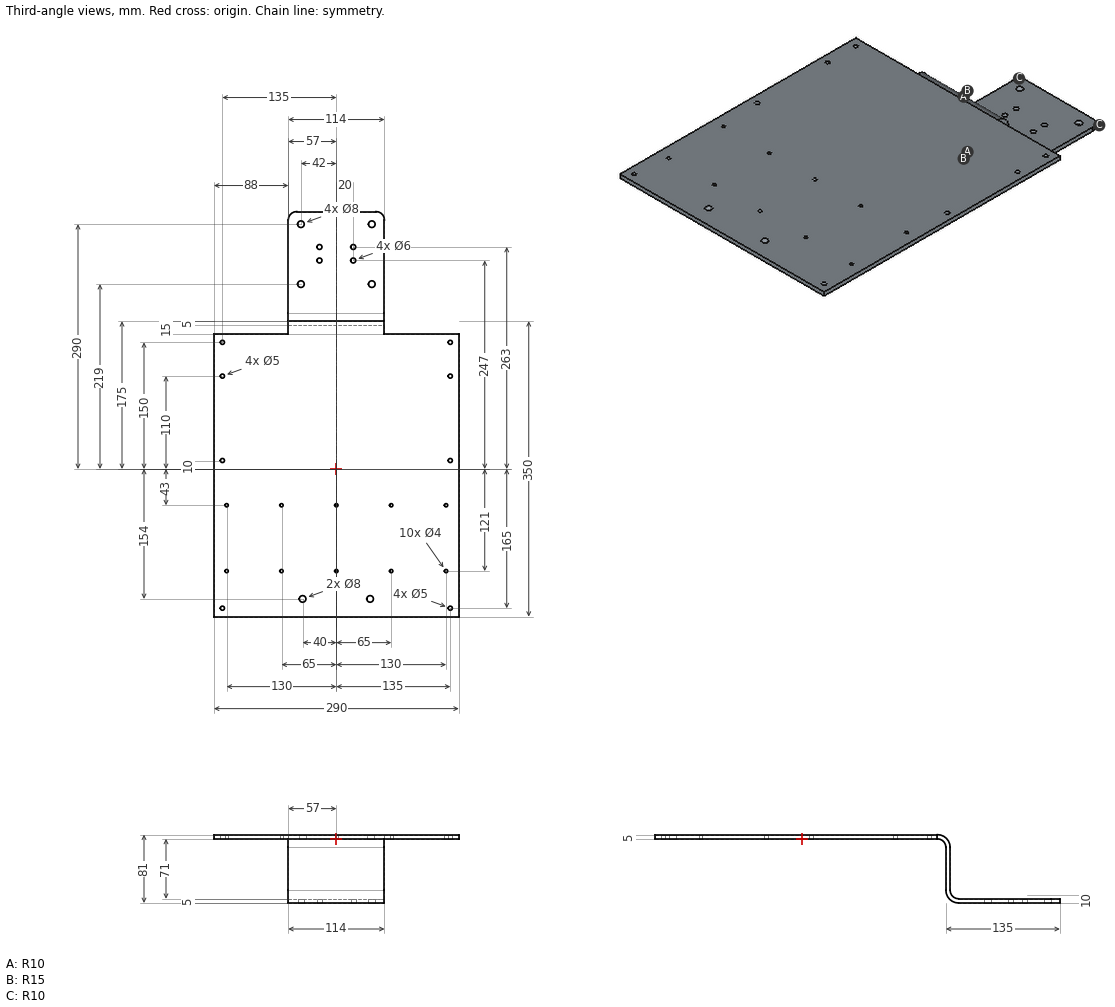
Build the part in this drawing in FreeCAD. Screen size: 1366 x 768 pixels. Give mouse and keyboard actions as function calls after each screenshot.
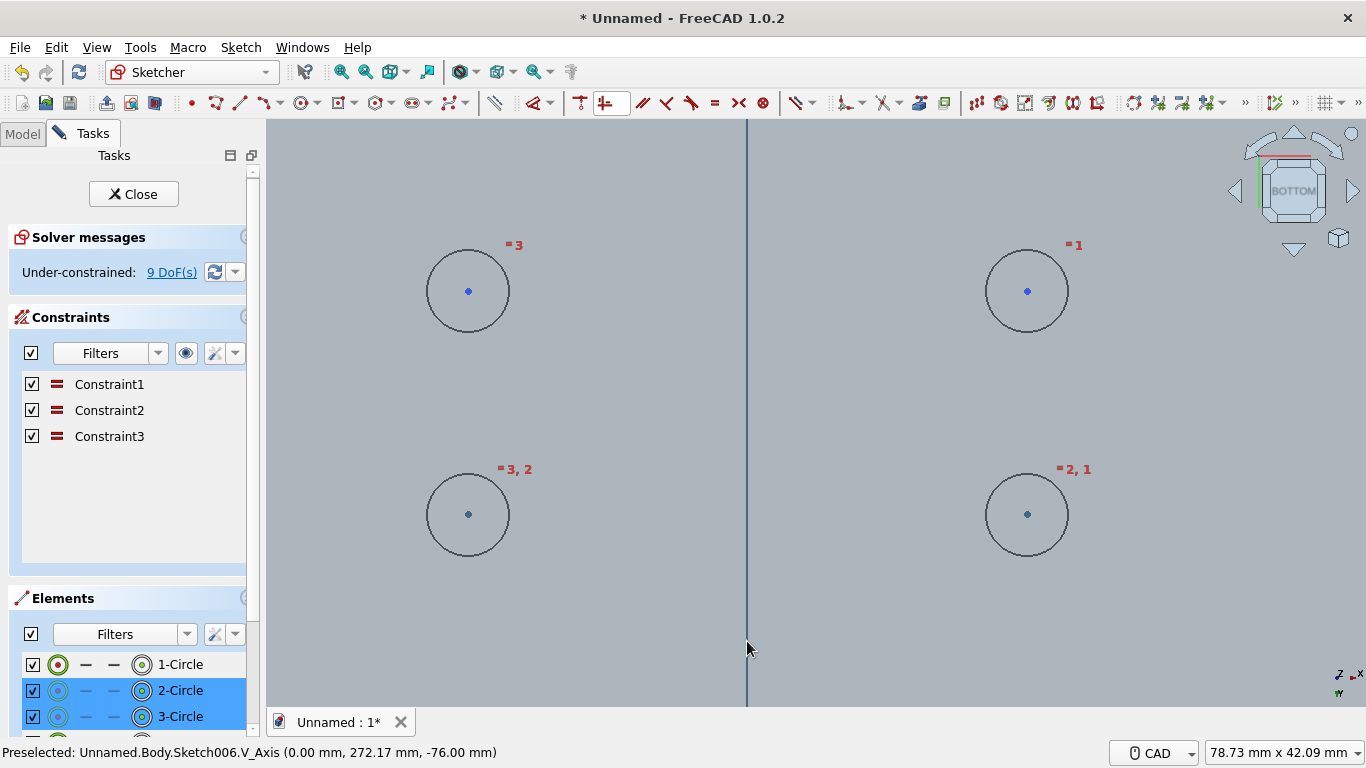
click(740, 104)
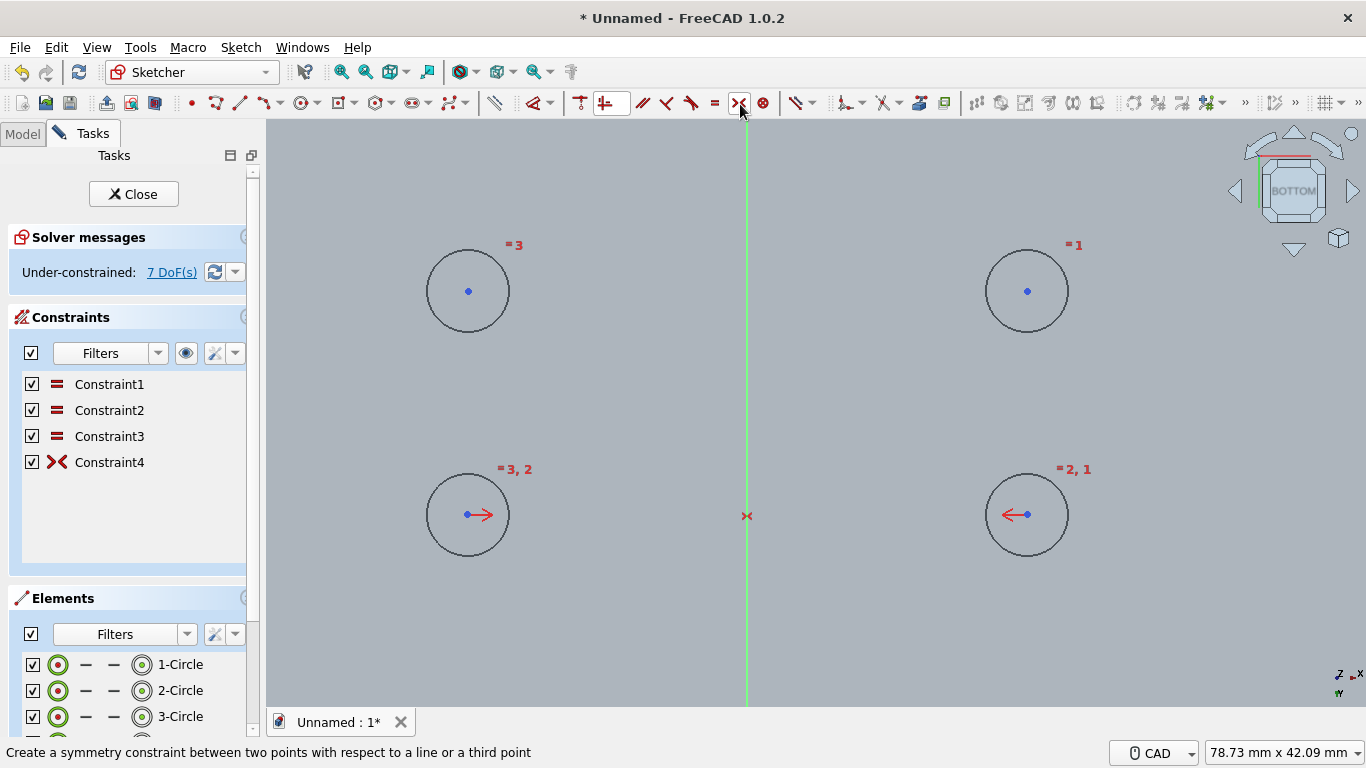
click(1027, 291)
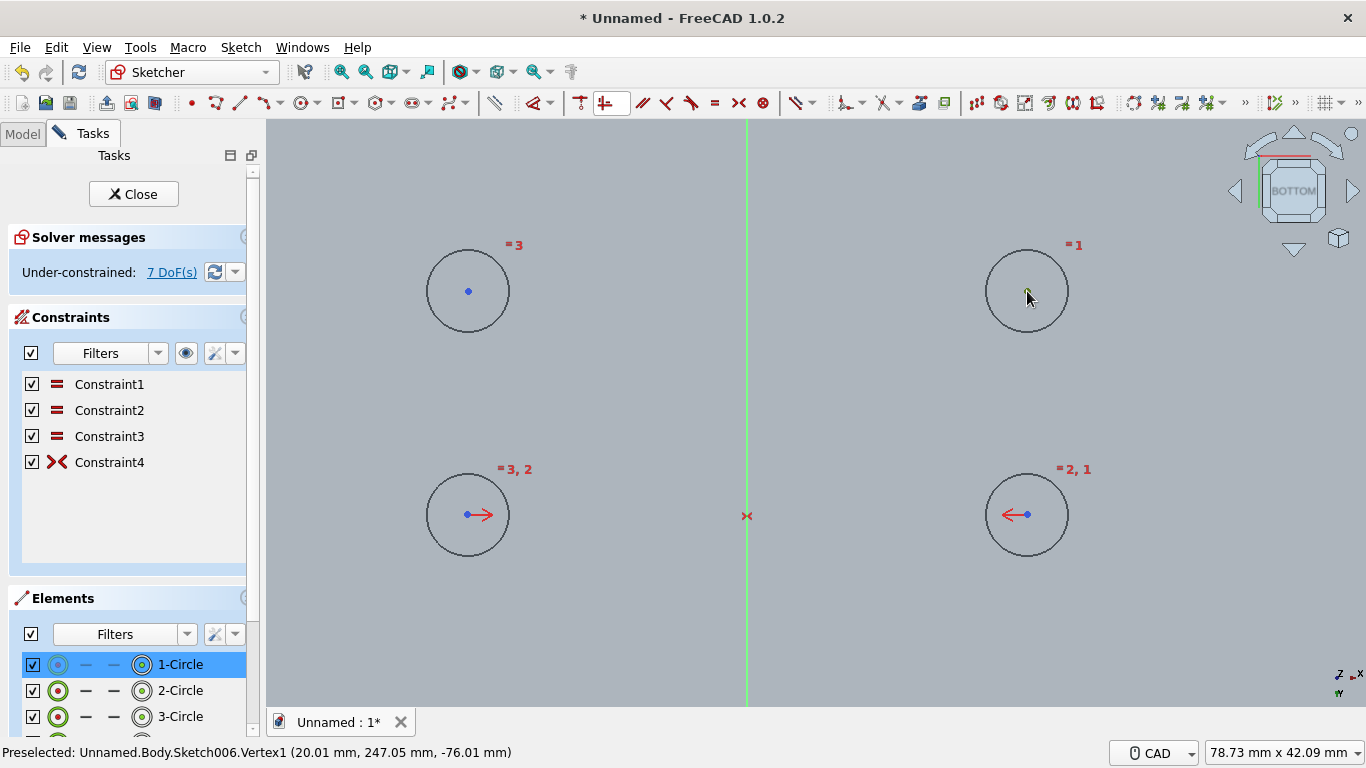
click(468, 291)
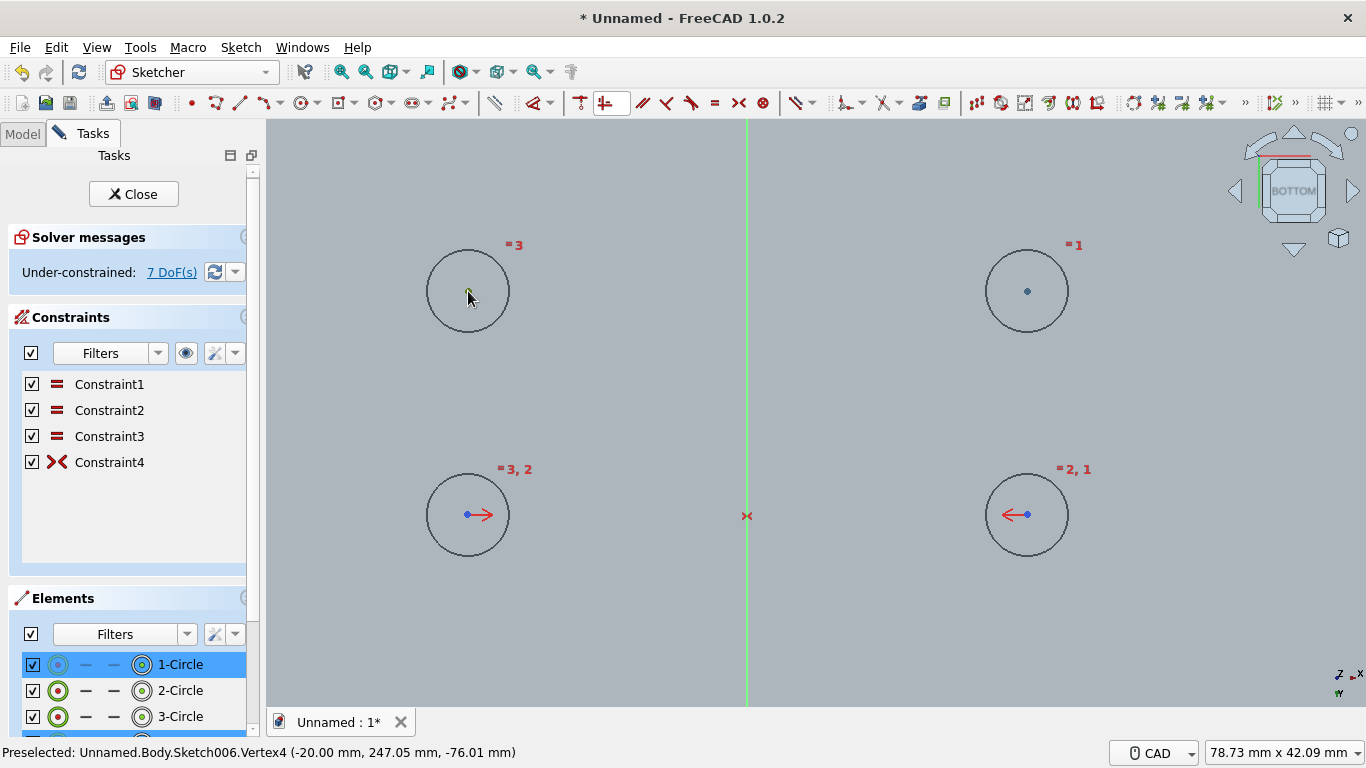
click(747, 641)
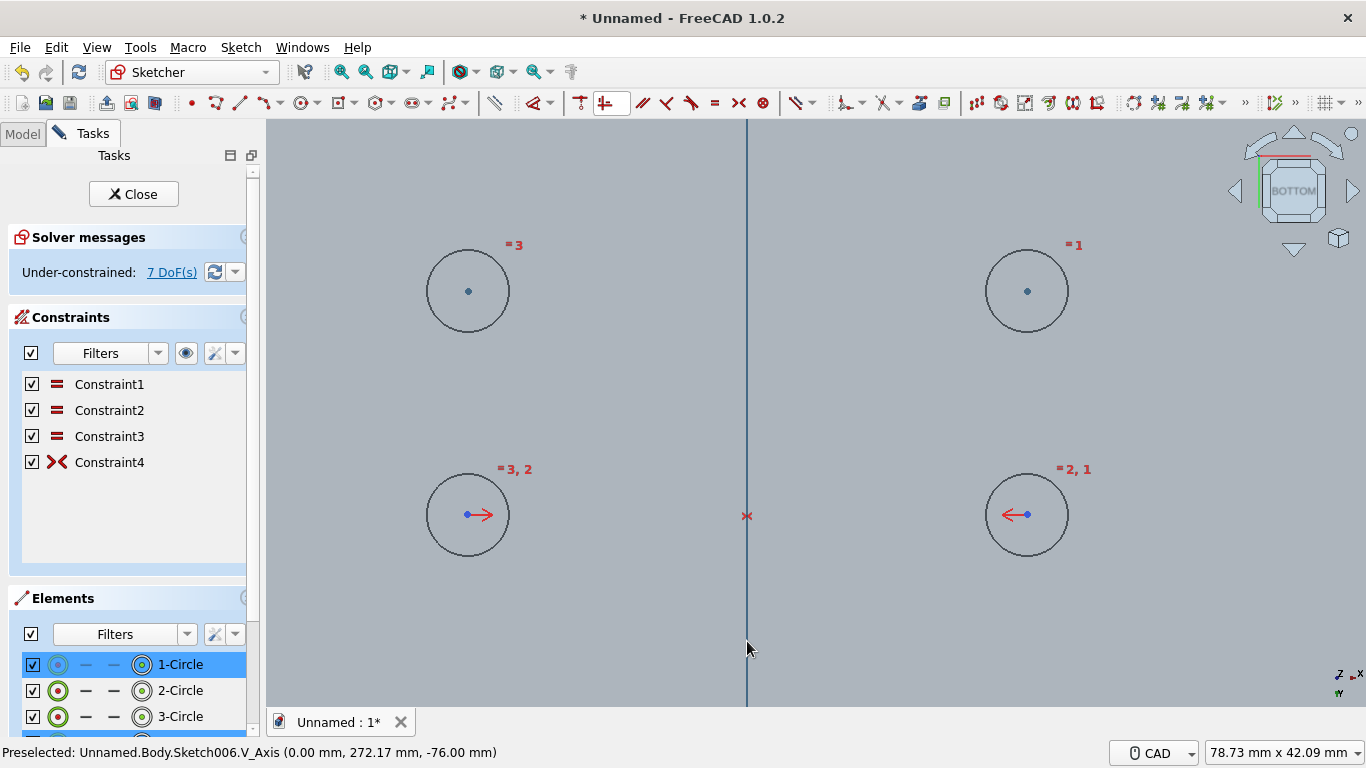
click(740, 104)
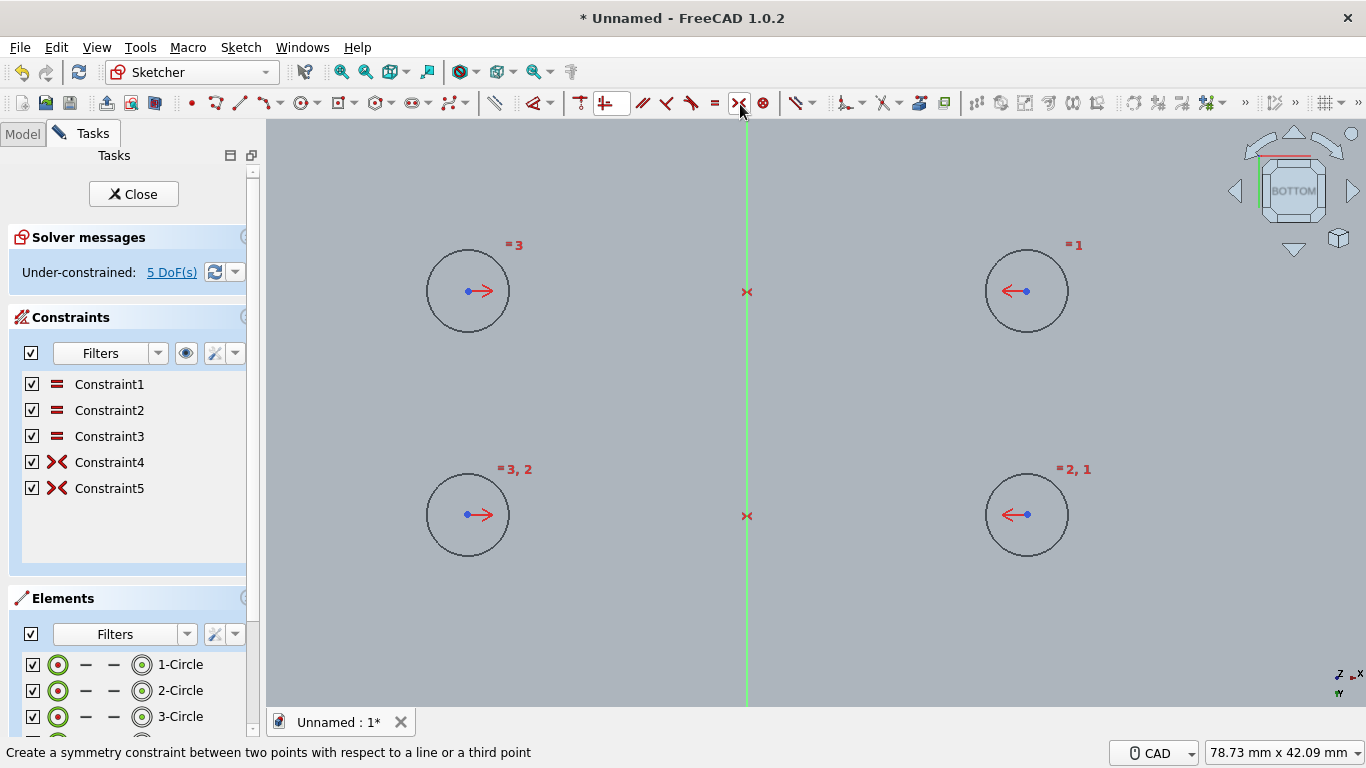
click(534, 104)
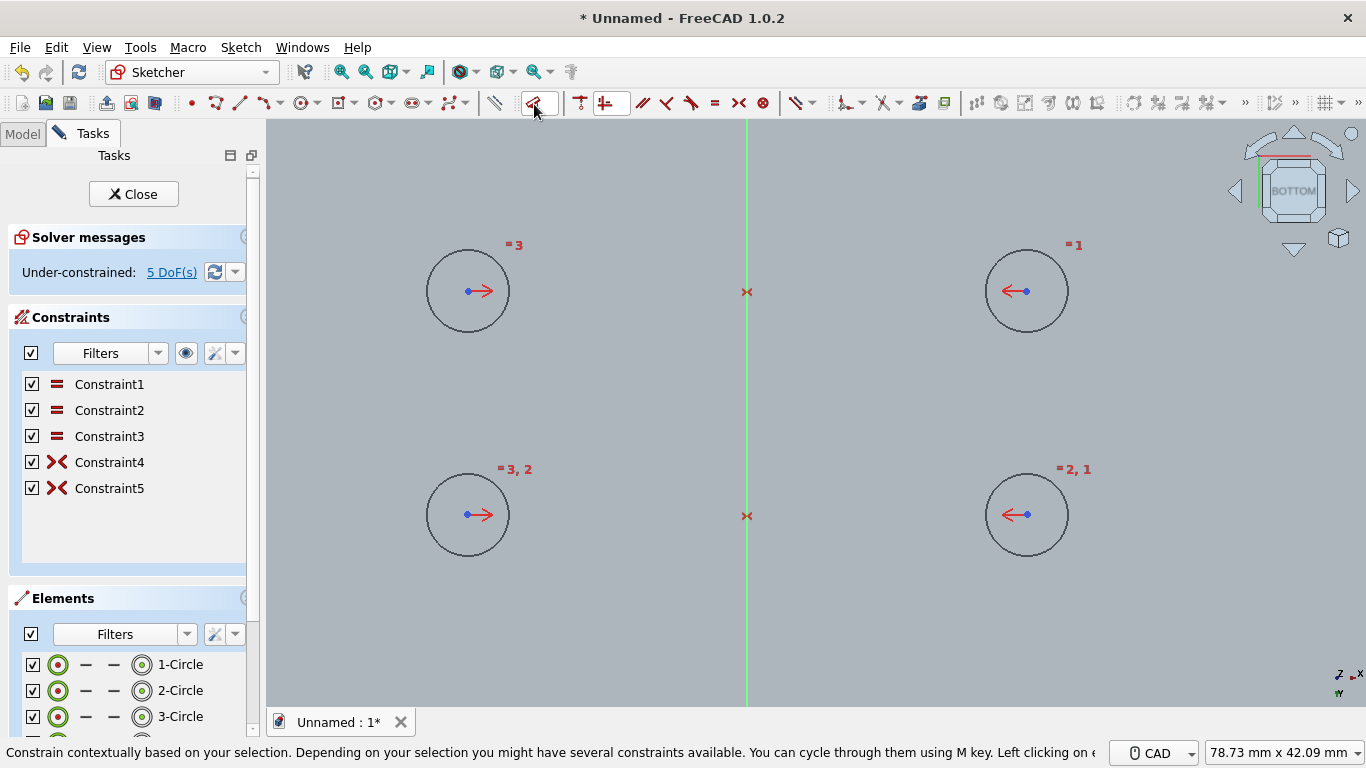
click(1056, 262)
click(1079, 239)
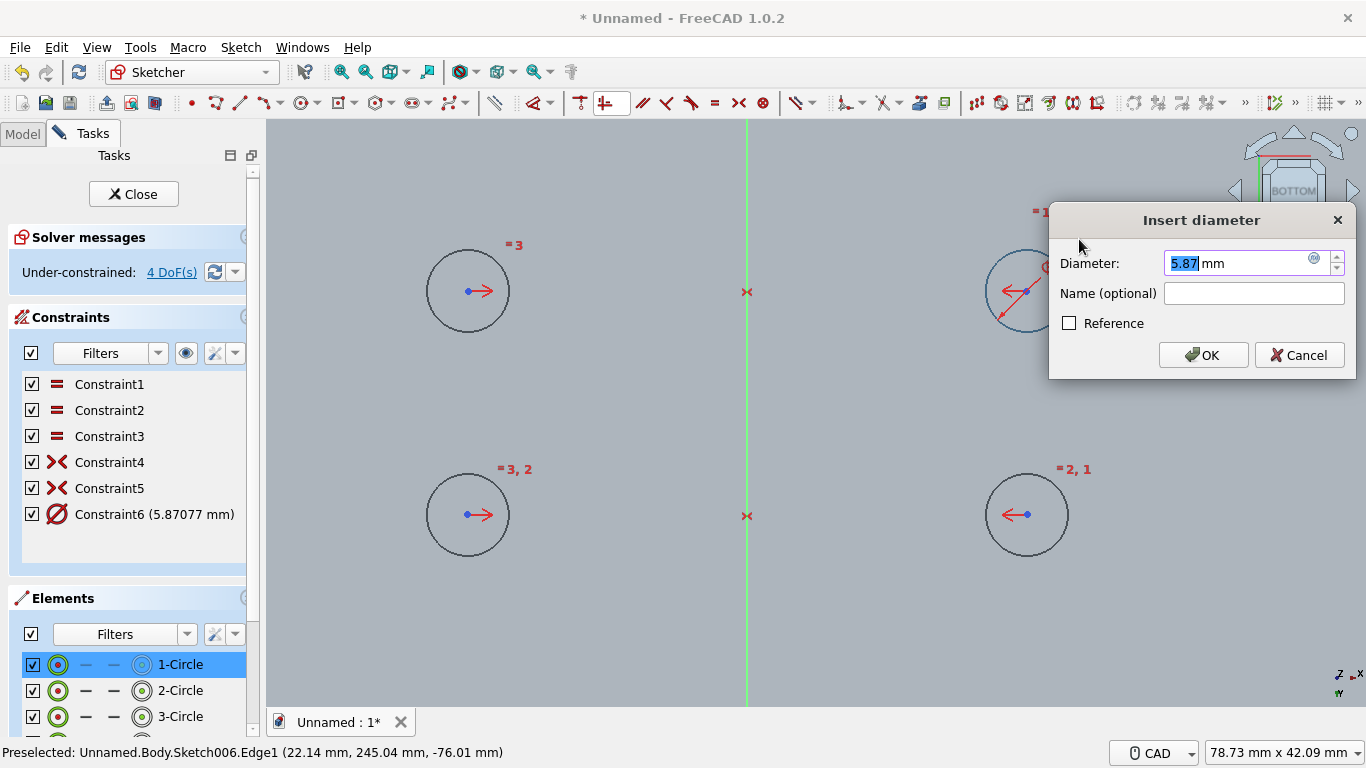
text(6)
key(Return)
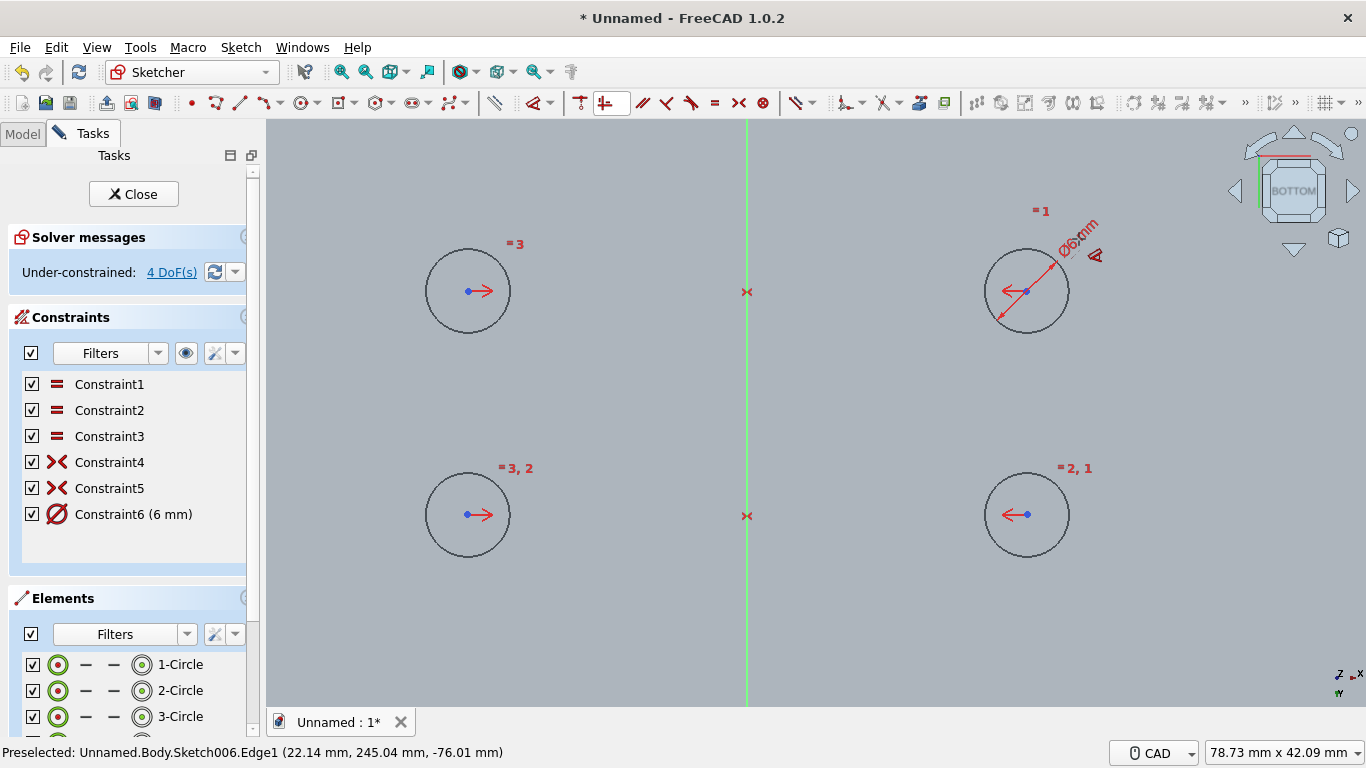
click(1027, 291)
click(887, 325)